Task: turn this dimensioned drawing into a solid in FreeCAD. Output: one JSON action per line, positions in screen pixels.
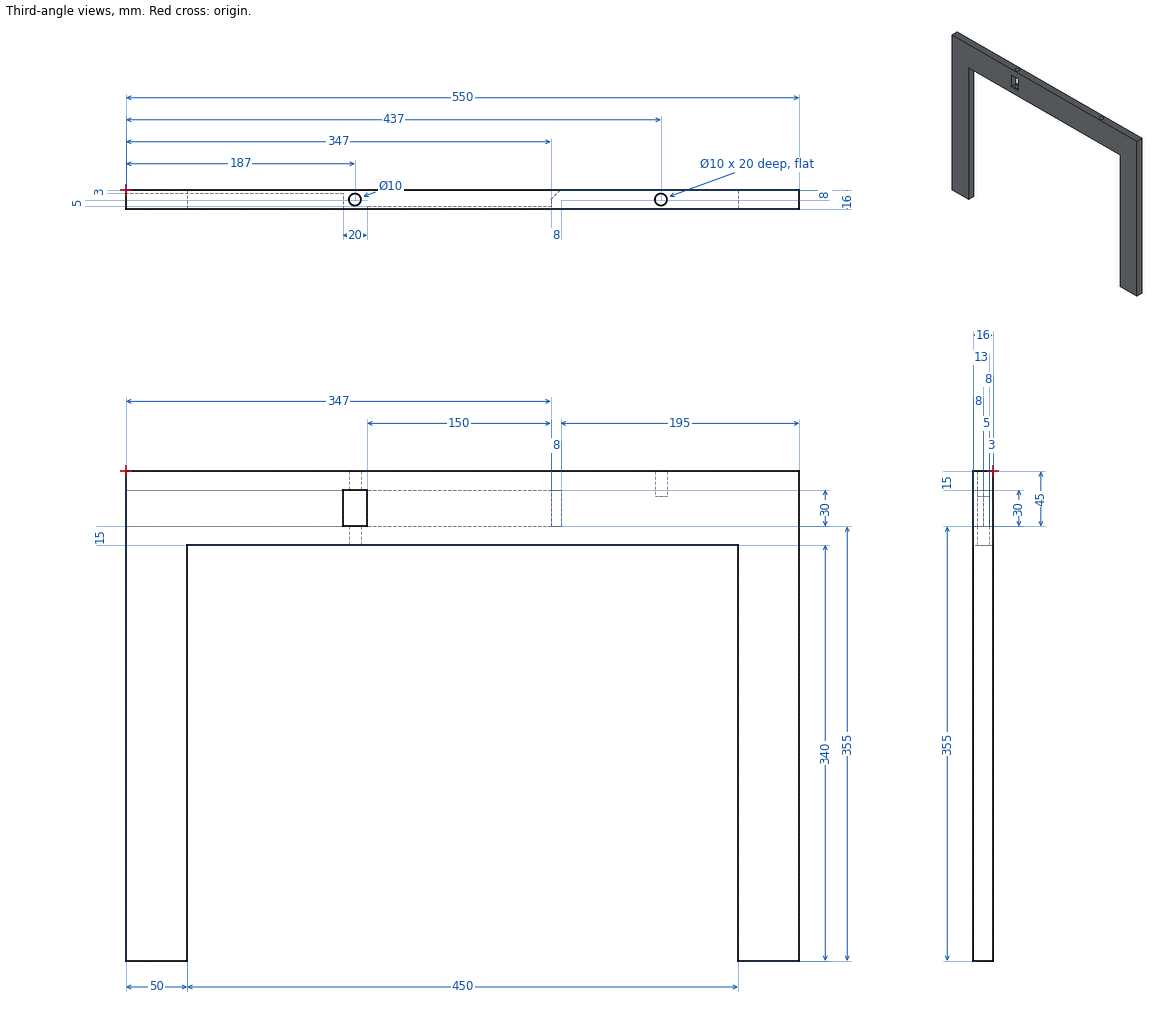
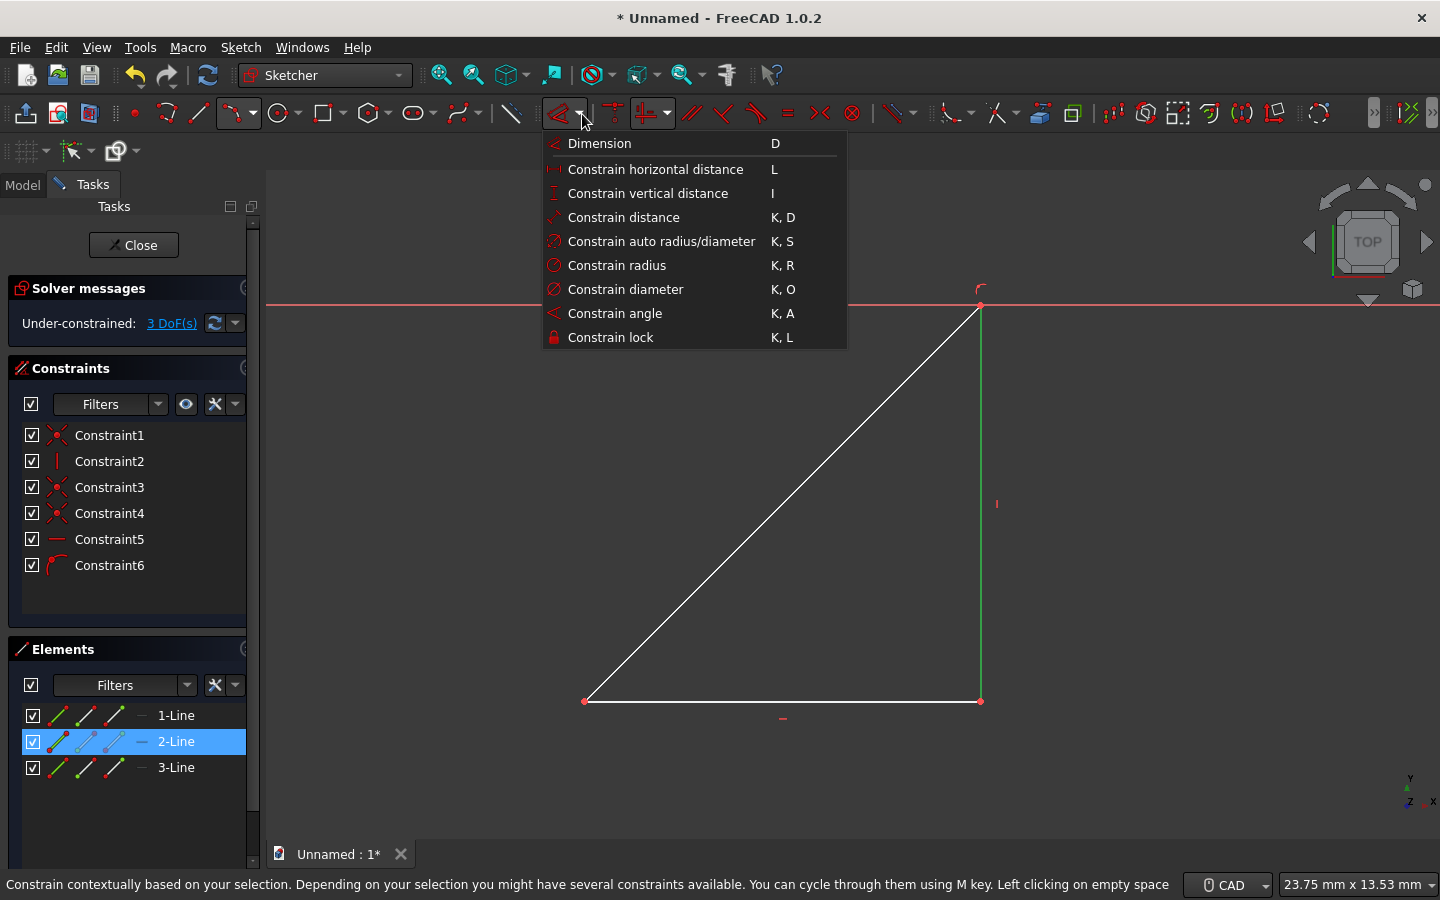
{"action": "left_click", "coordinate": [695, 193]}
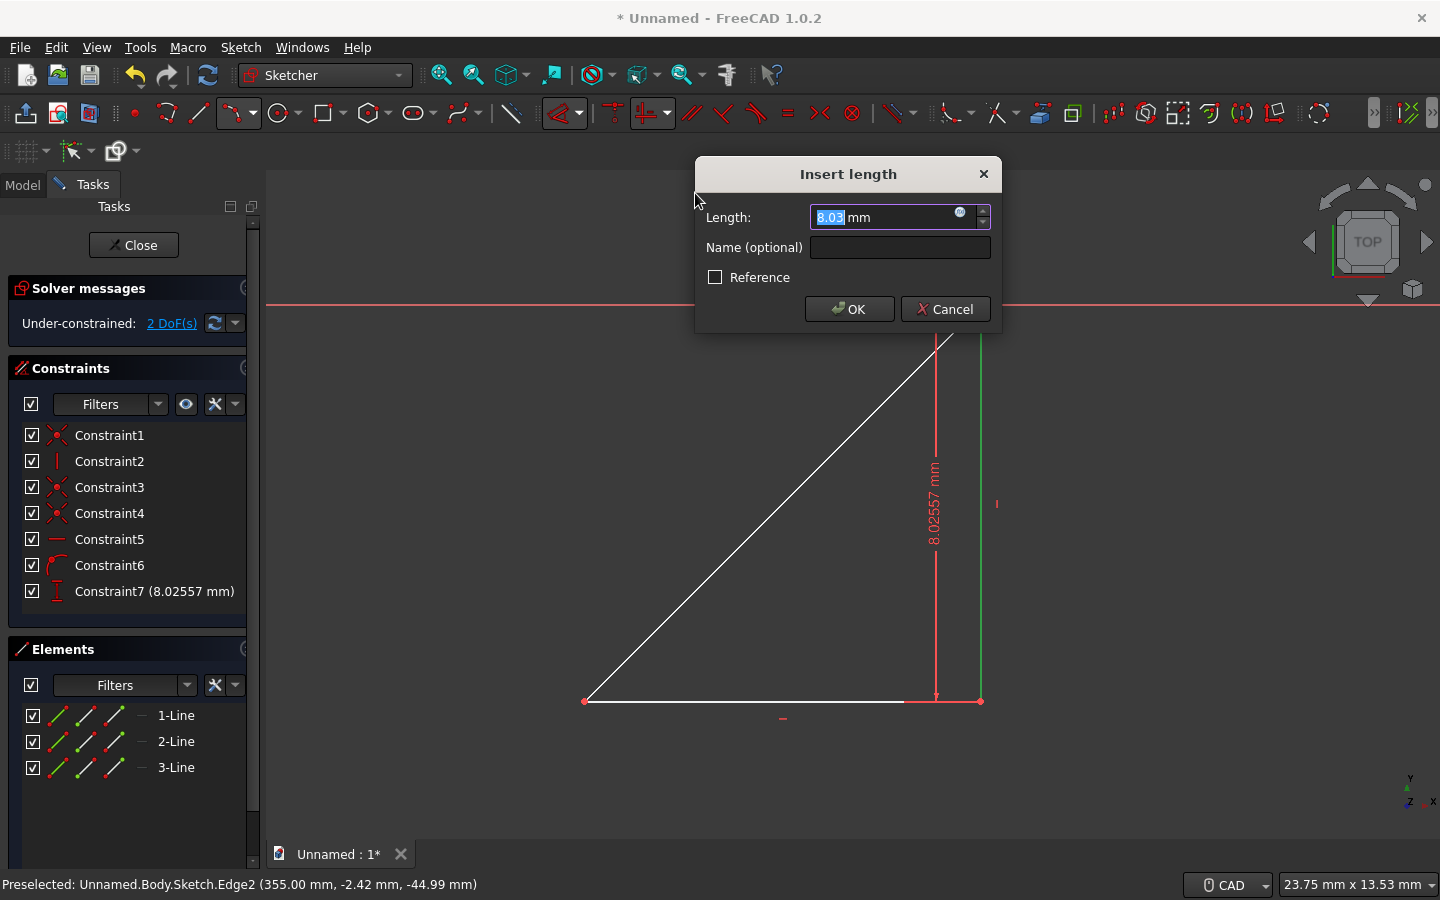
{"action": "type", "text": "8"}
{"action": "key", "text": "Return"}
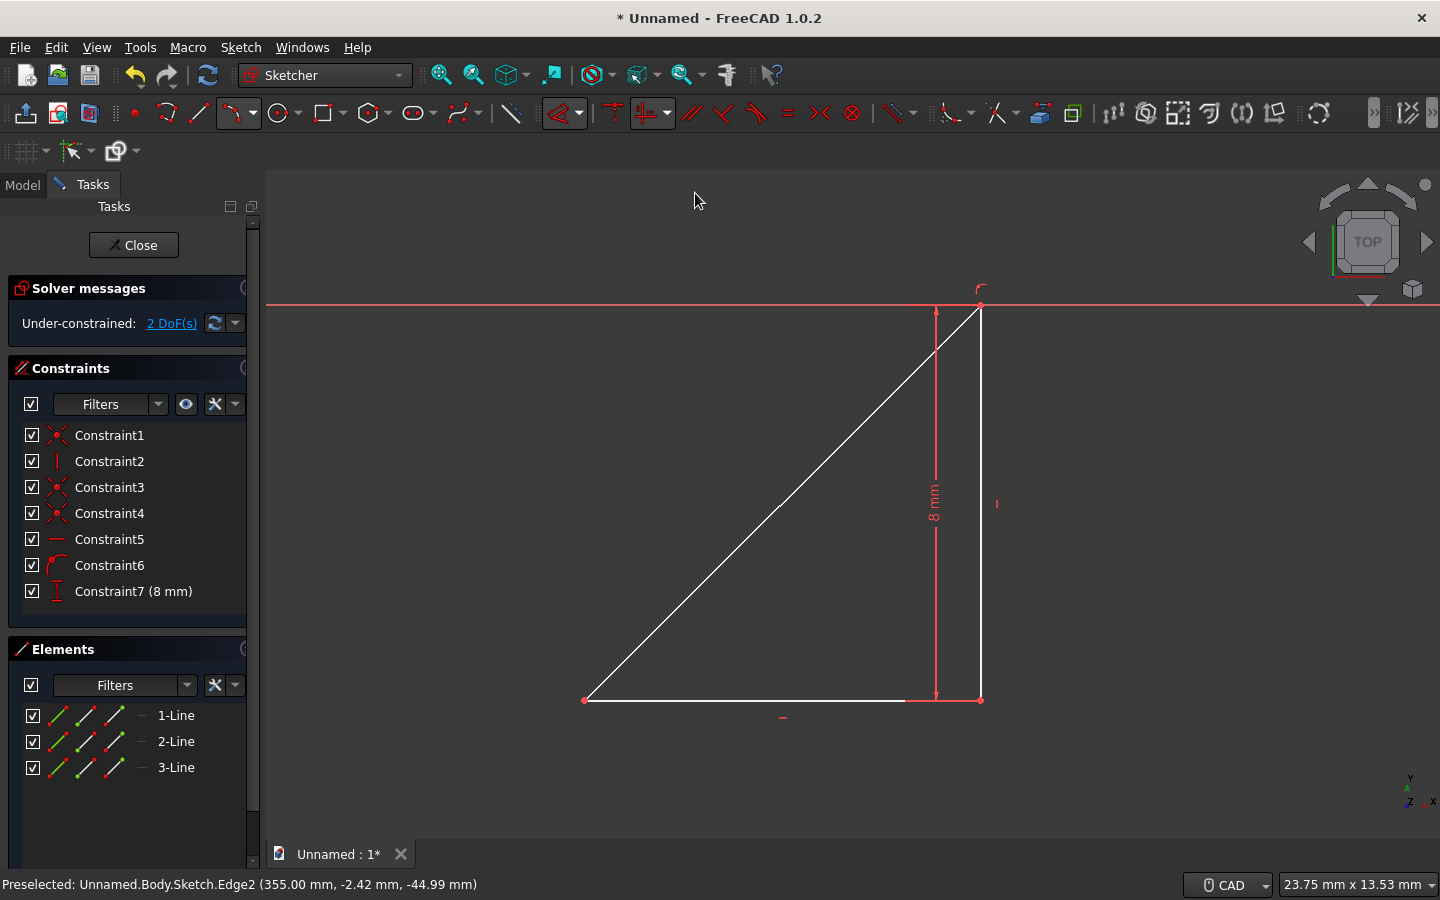
{"action": "left_click", "coordinate": [862, 701]}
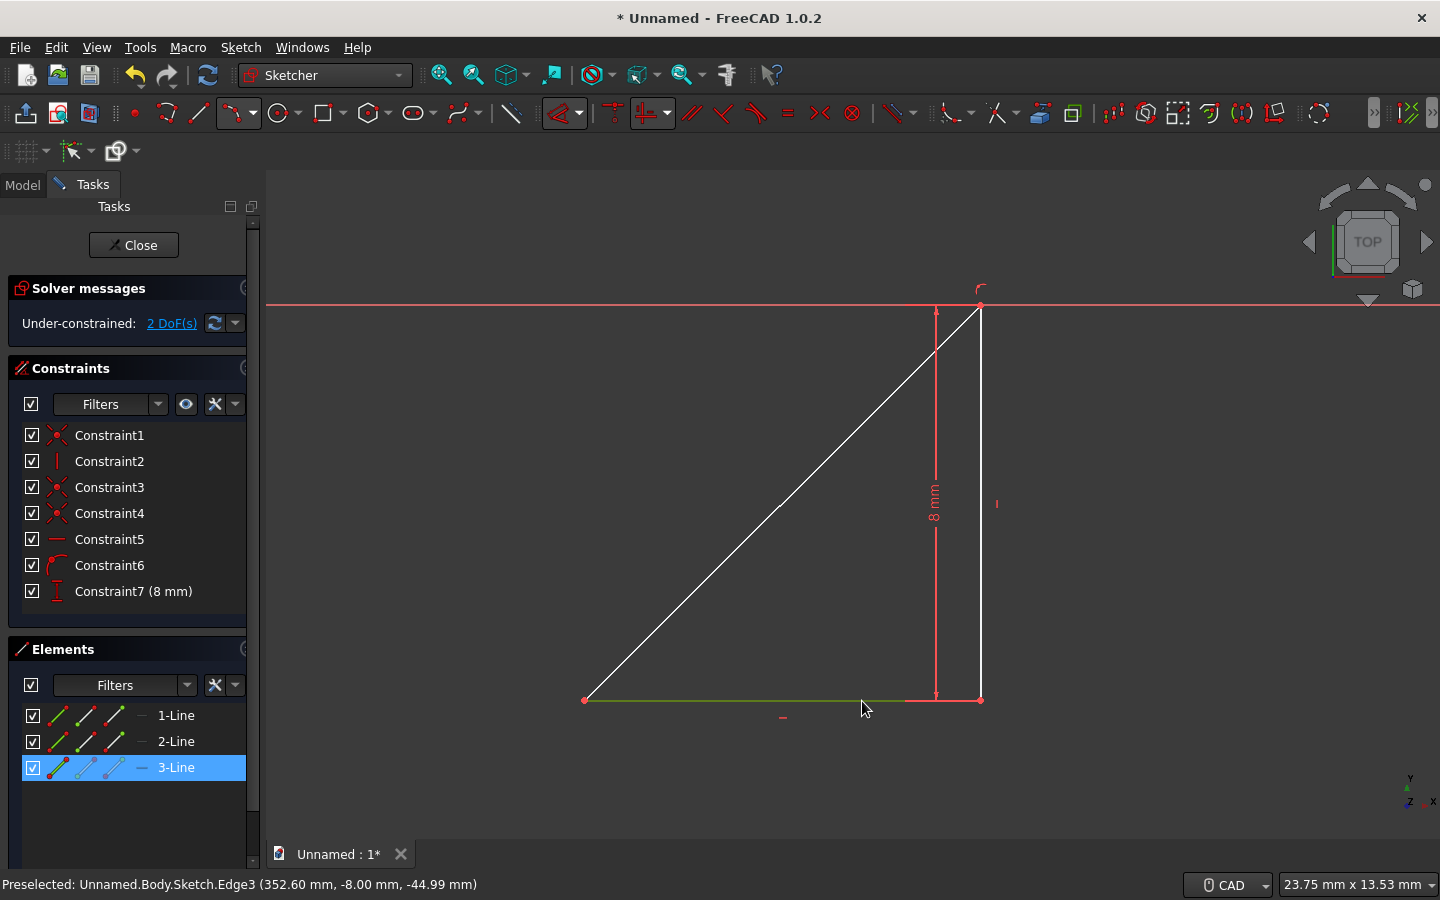
{"action": "key", "text": "l"}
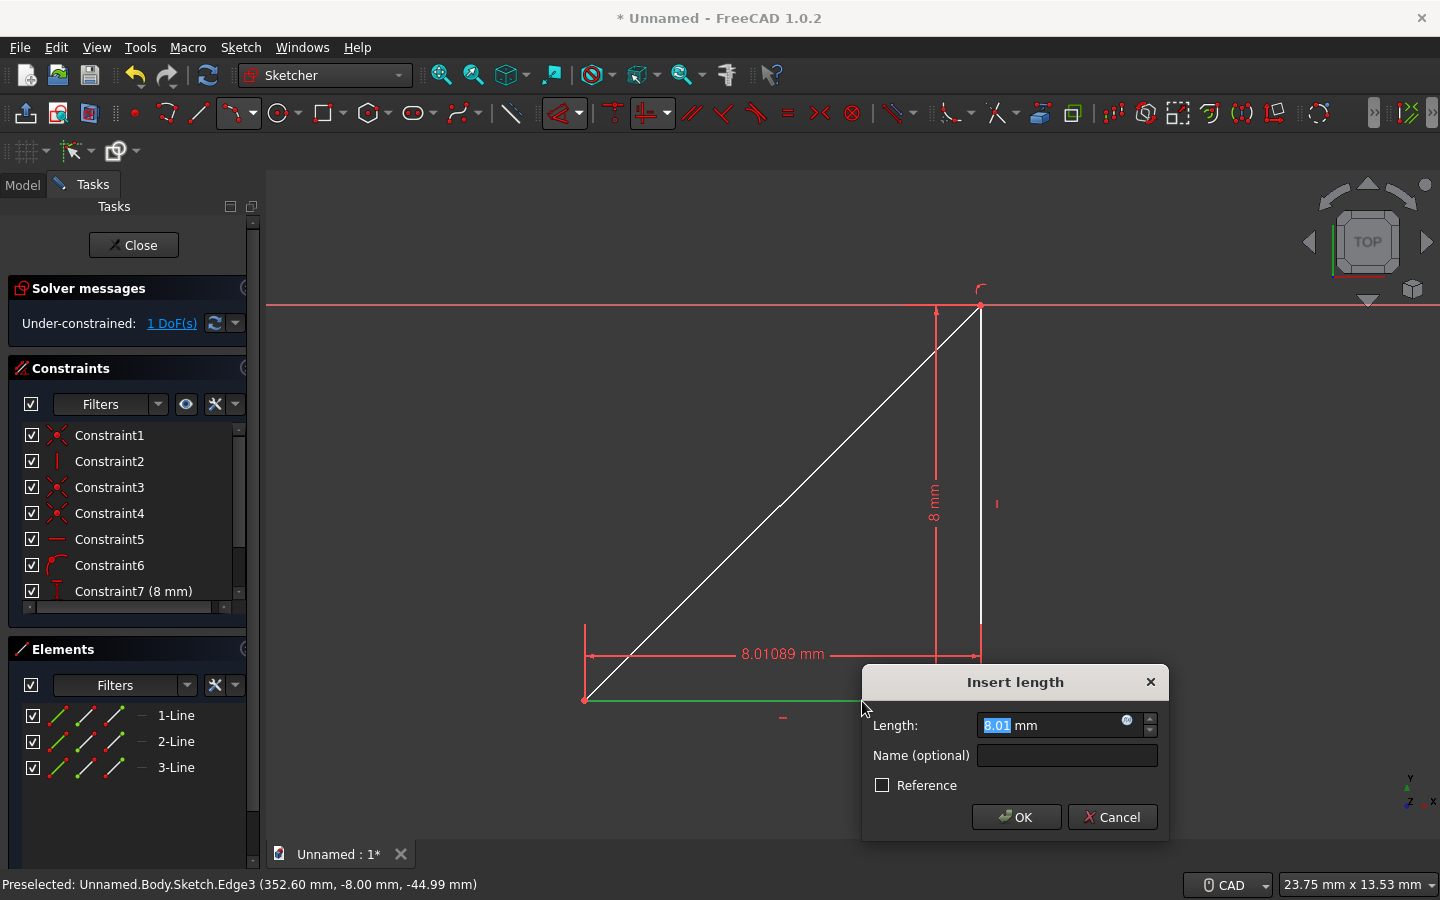
{"action": "type", "text": "8"}
{"action": "key", "text": "Return"}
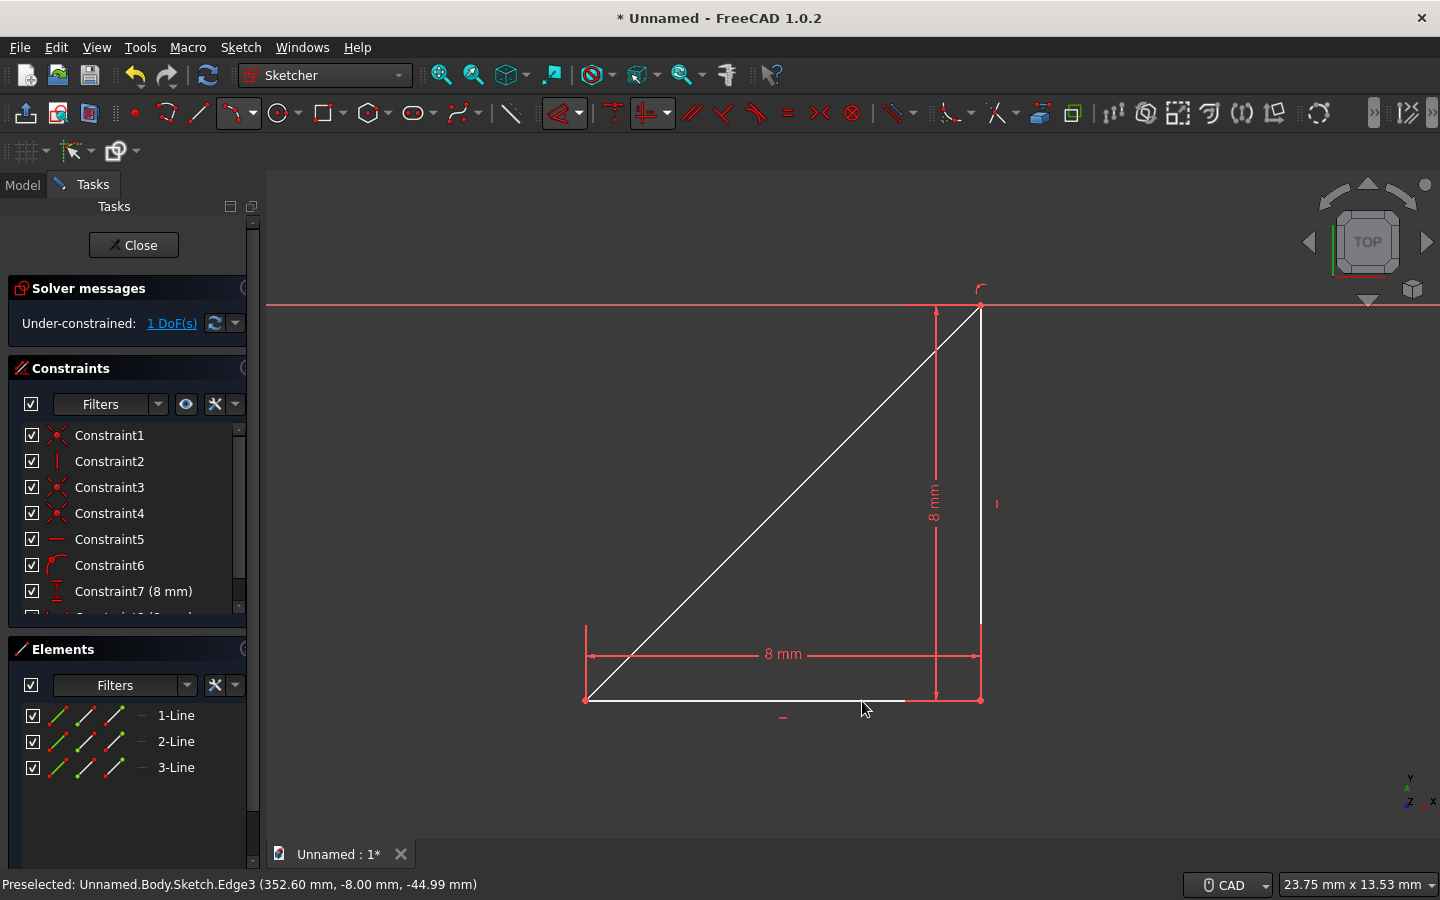
{"action": "left_click", "coordinate": [586, 701]}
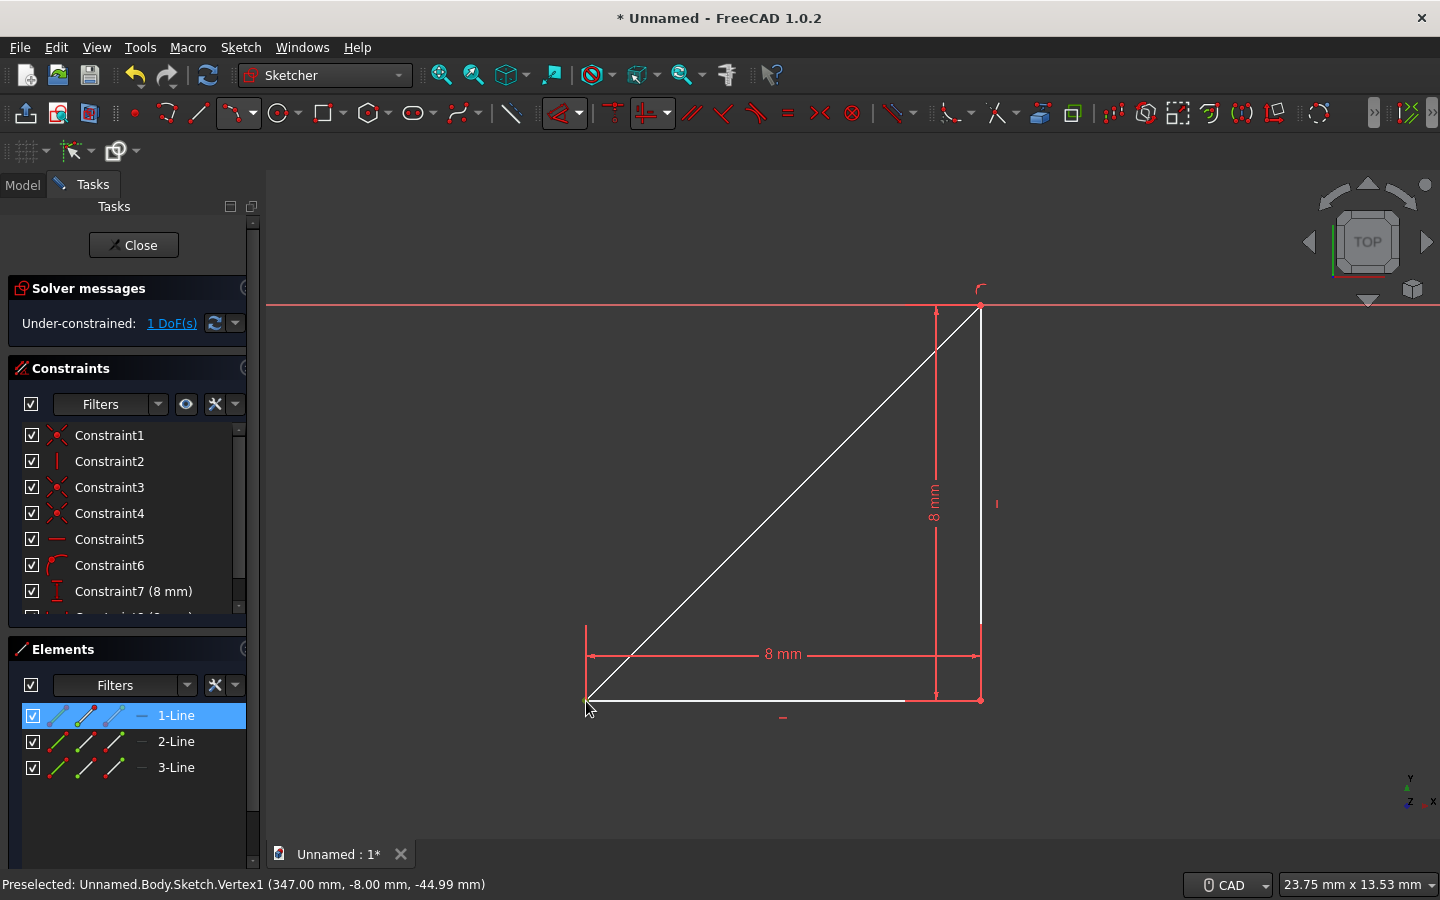
{"action": "left_click", "coordinate": [582, 114]}